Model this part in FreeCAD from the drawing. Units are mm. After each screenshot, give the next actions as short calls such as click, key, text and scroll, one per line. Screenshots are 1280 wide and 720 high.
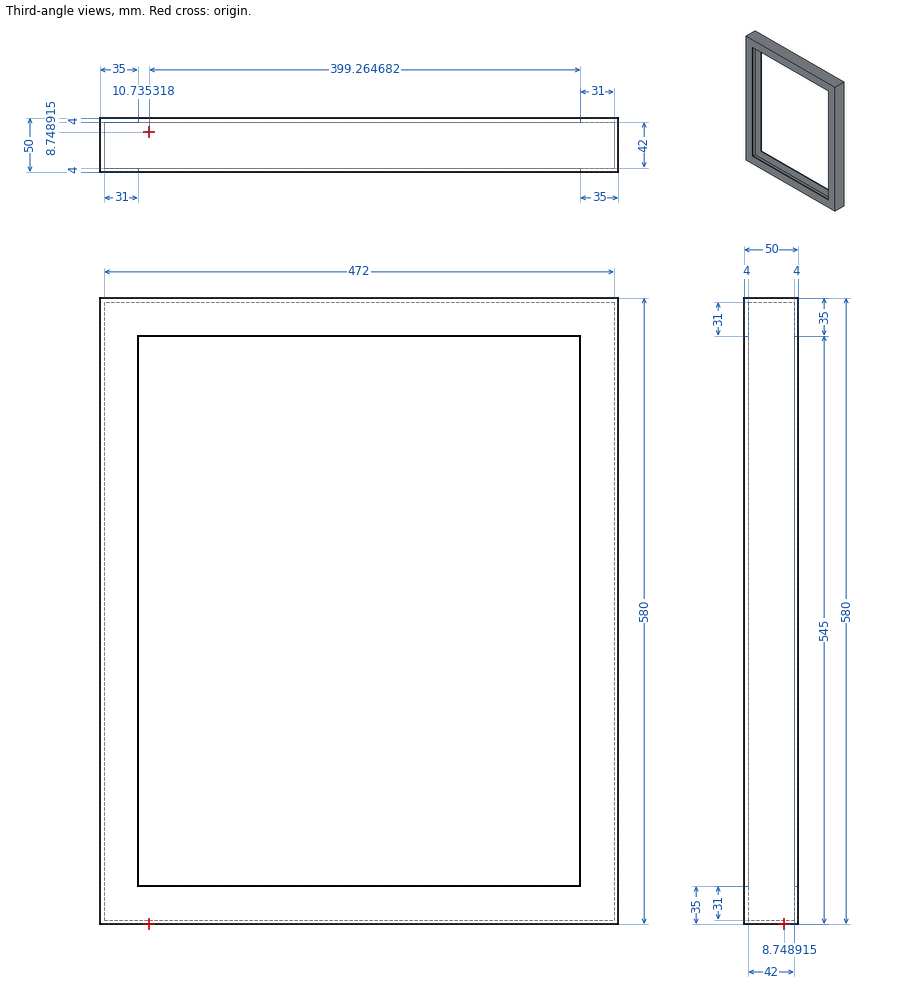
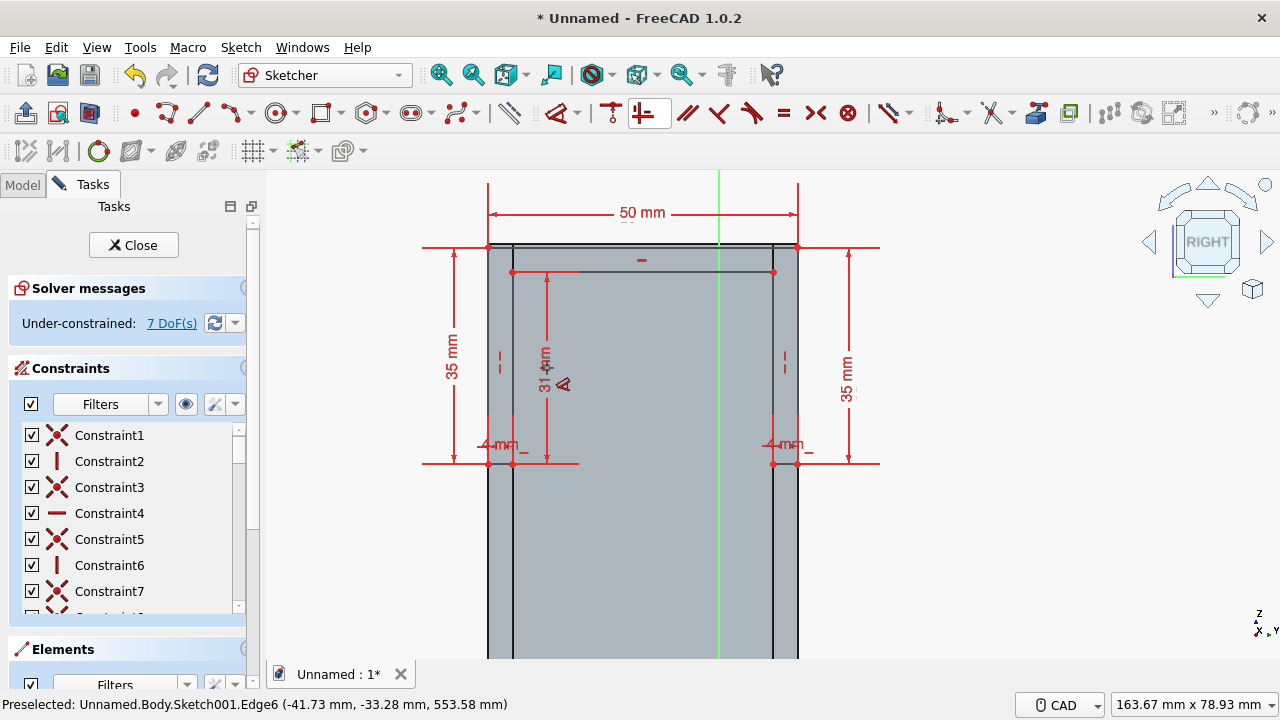
scroll(711, 252, down, 12)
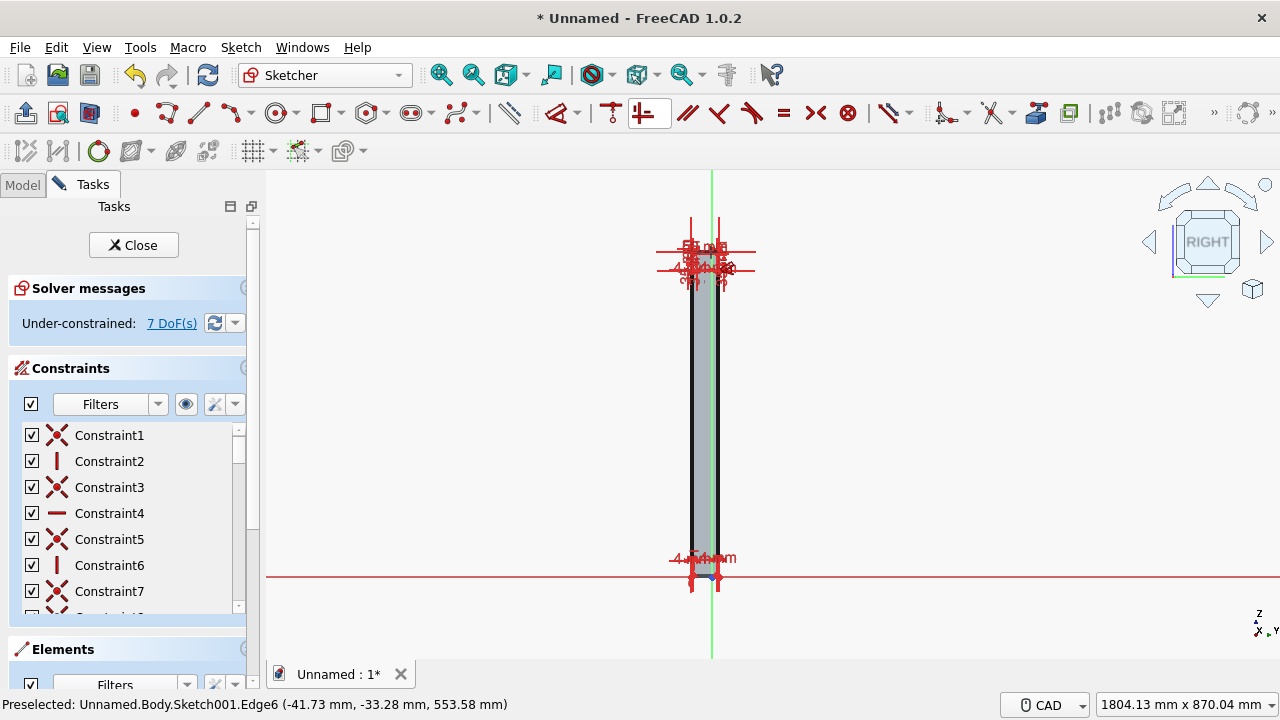
scroll(710, 575, up, 10)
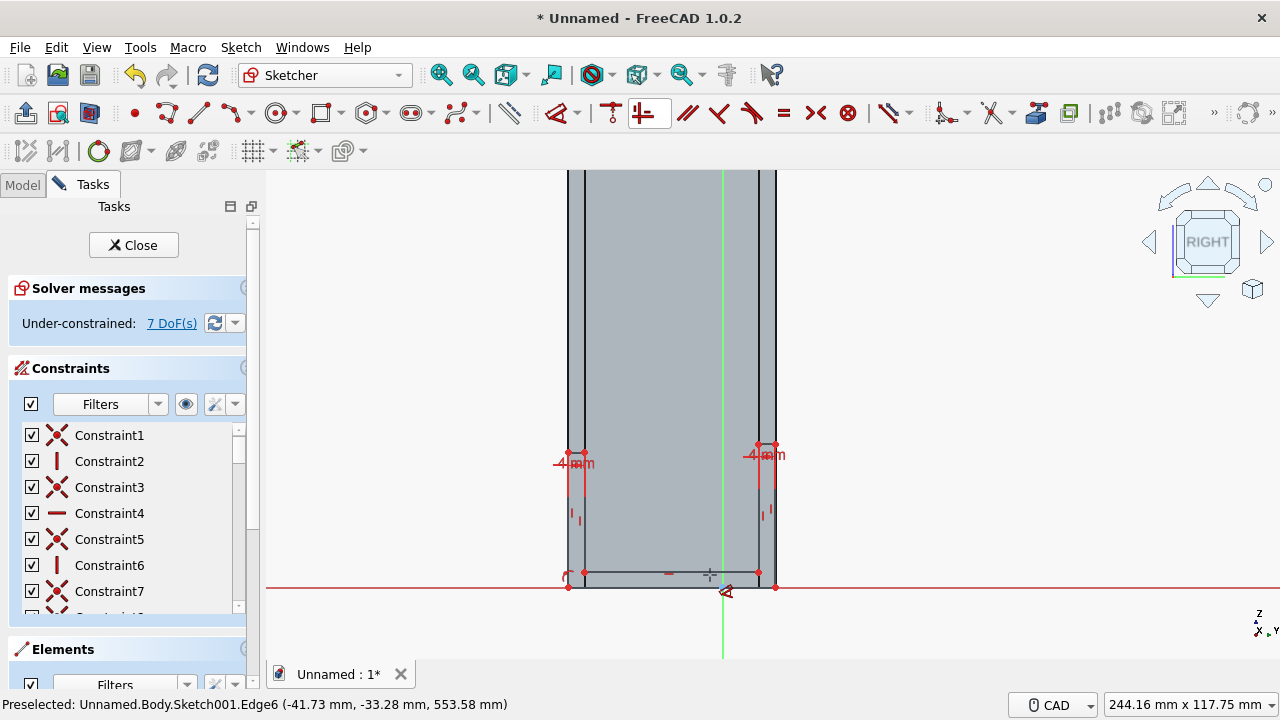
click(707, 572)
click(672, 606)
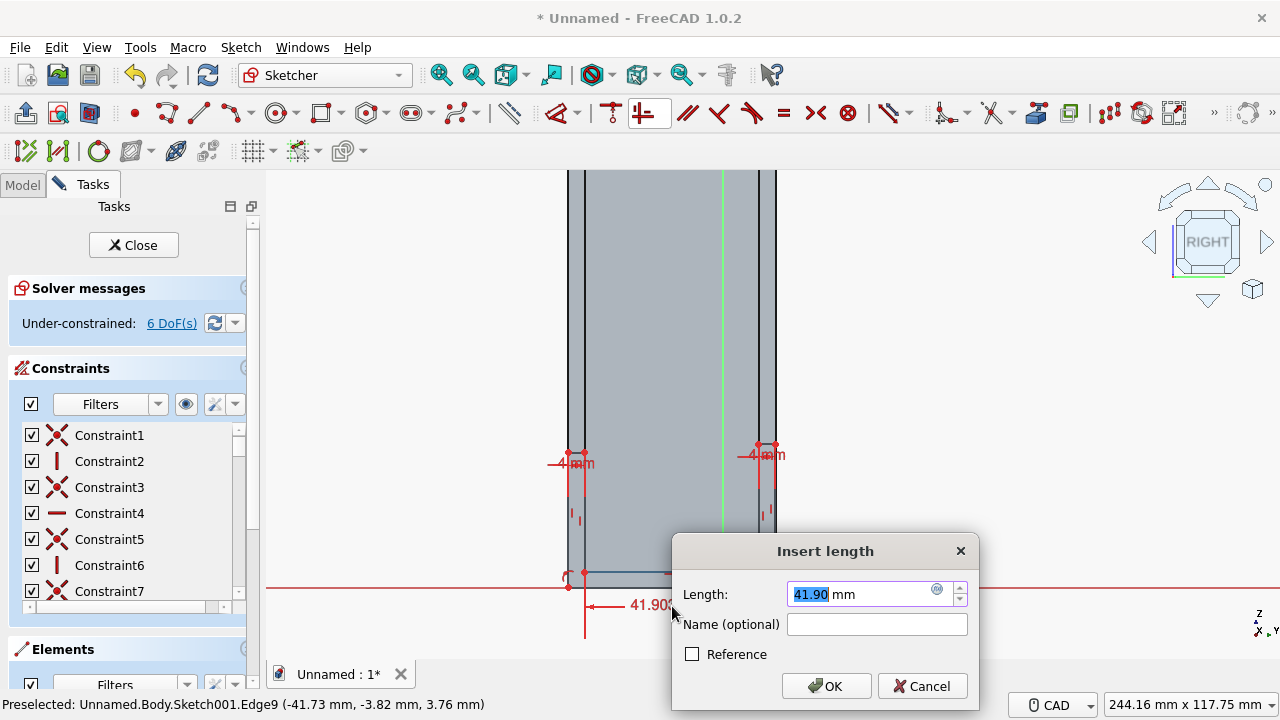
text(42)
key(Return)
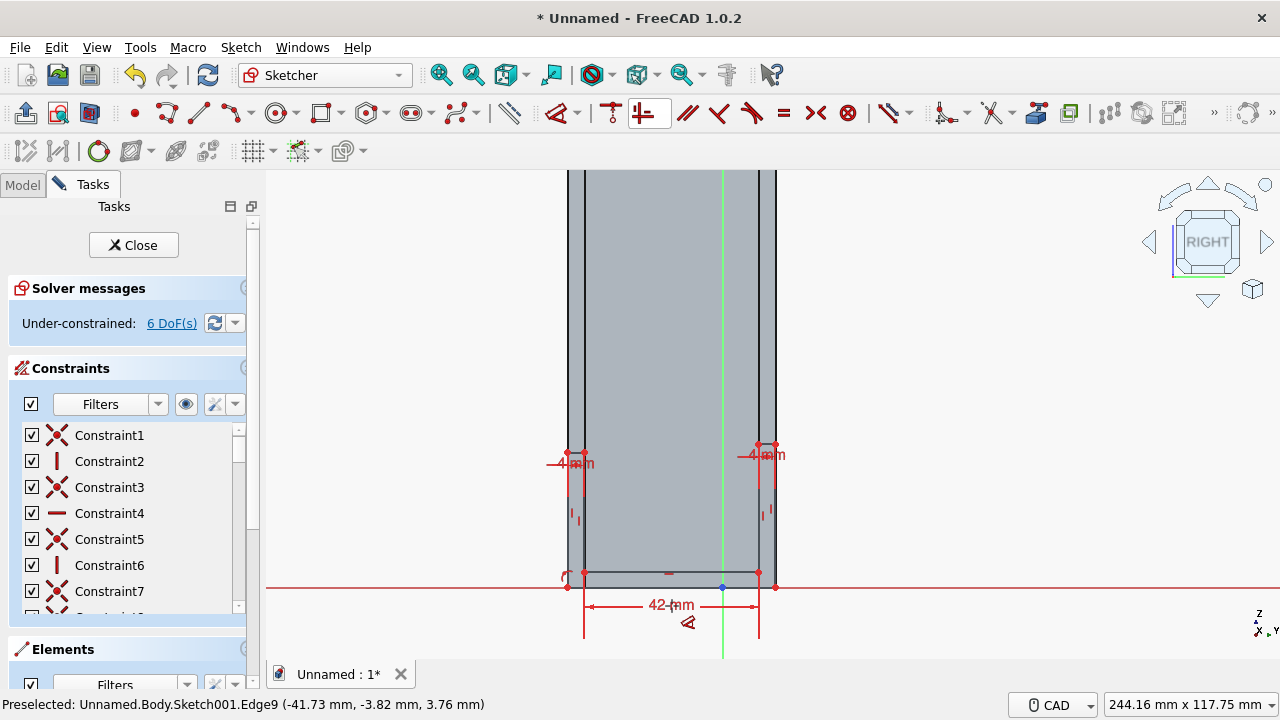
click(584, 536)
click(550, 512)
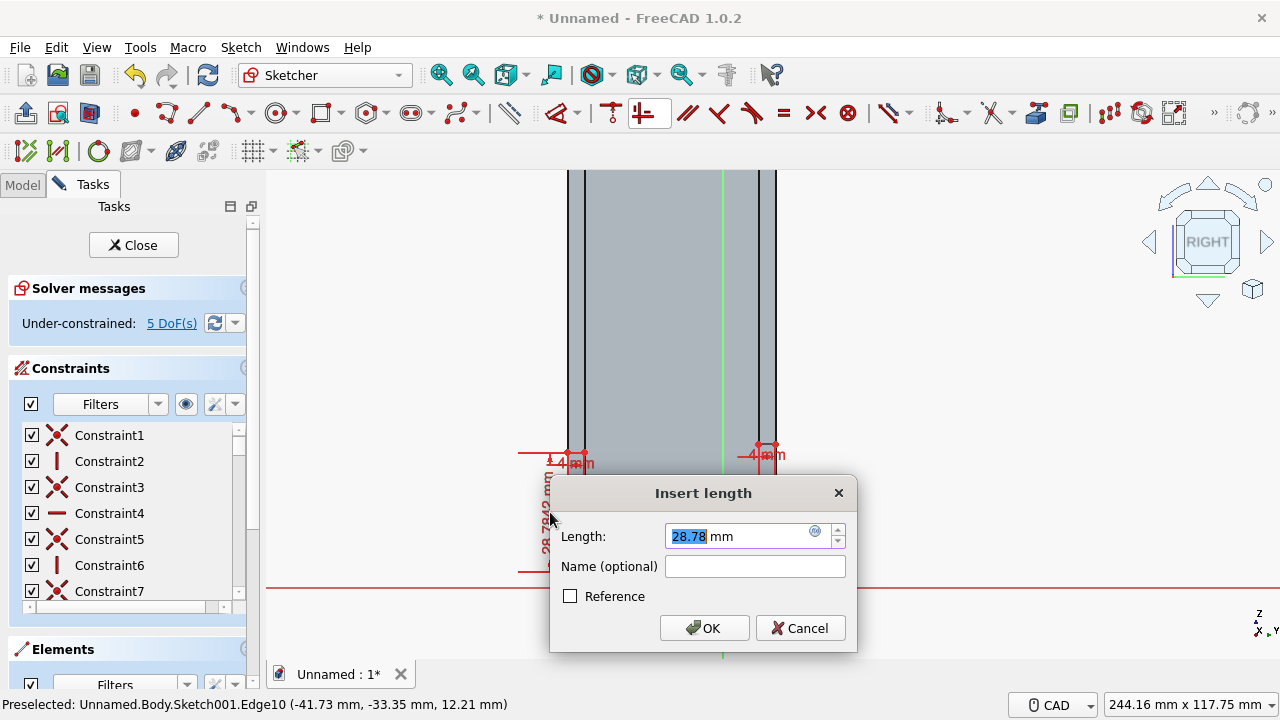
text(31)
key(Return)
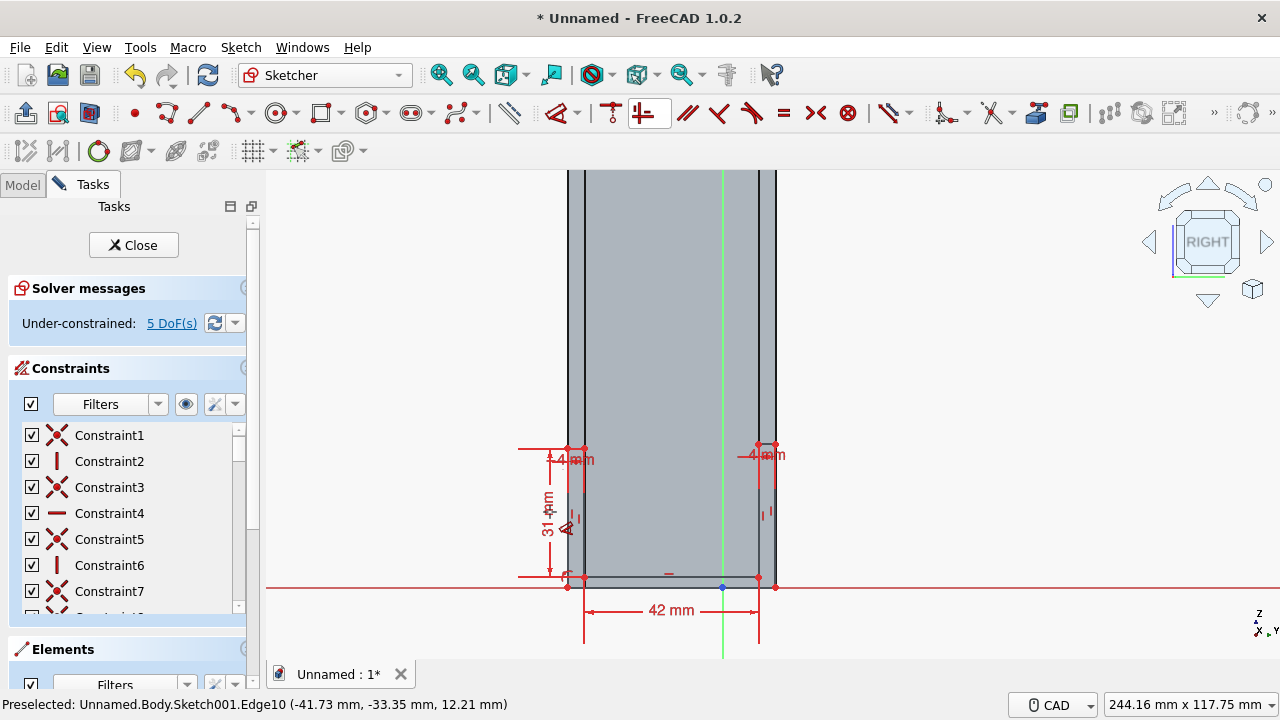
click(568, 490)
click(534, 486)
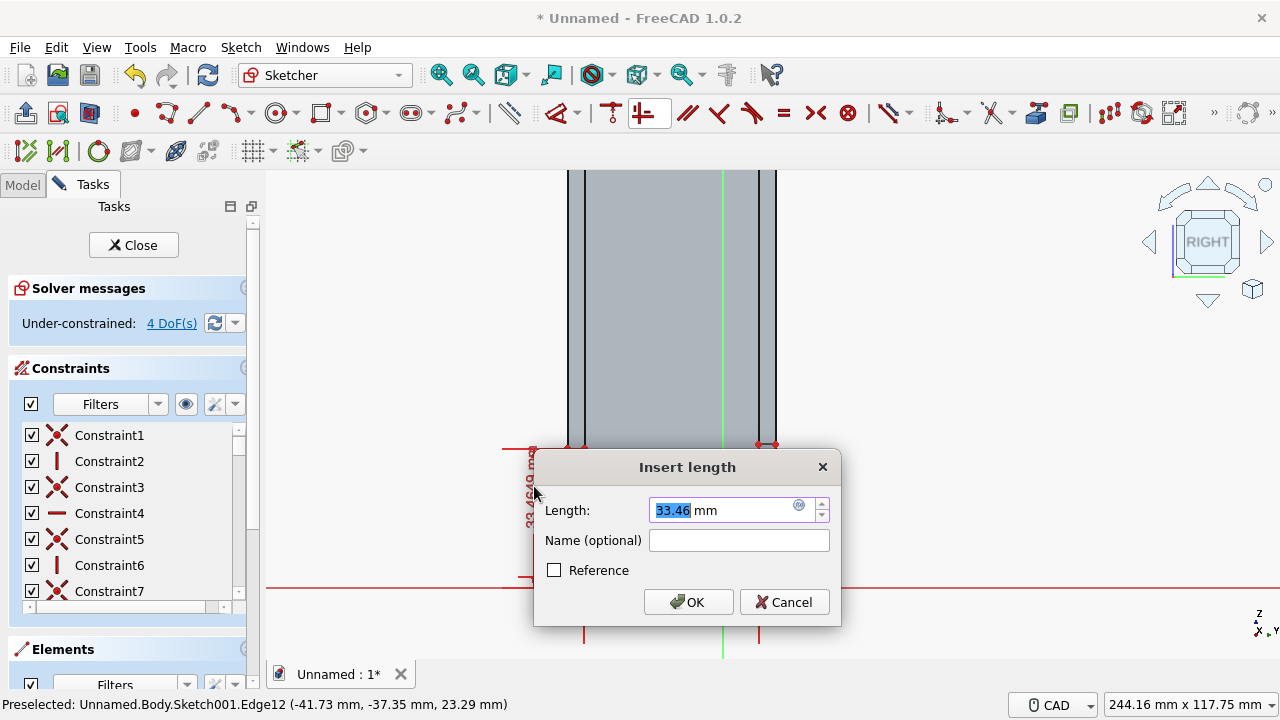
text(35)
key(Return)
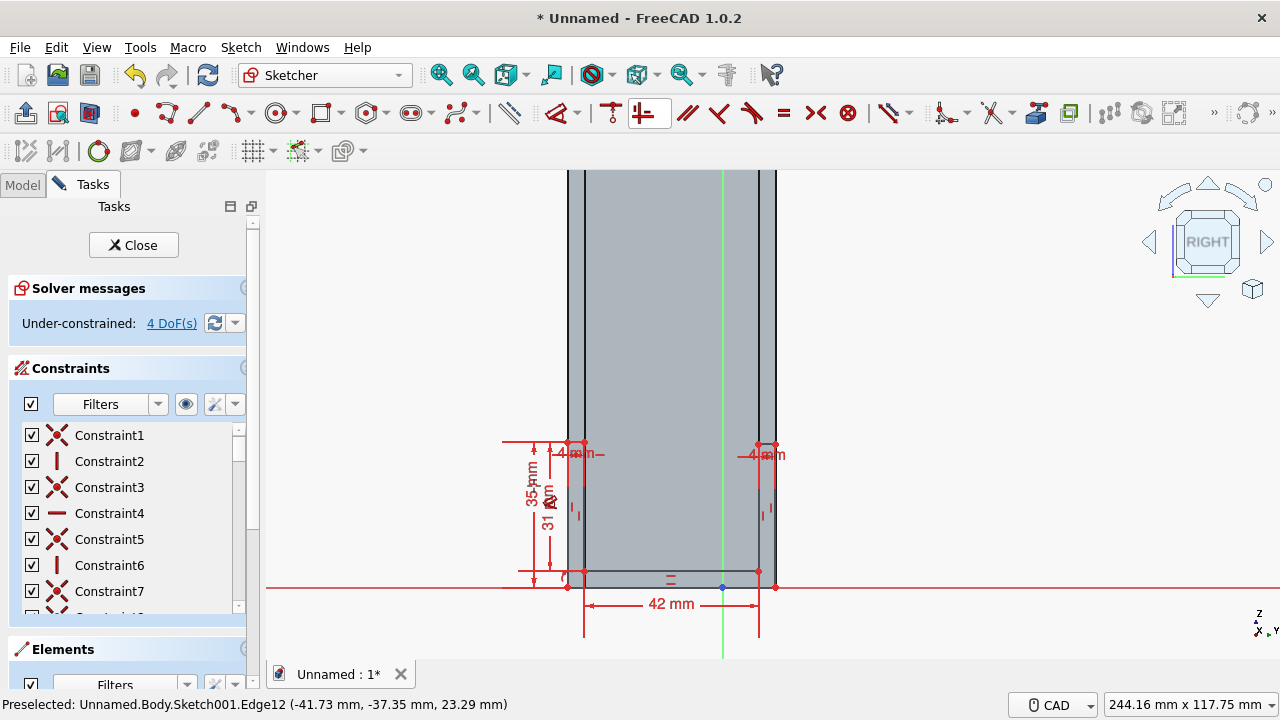
click(775, 545)
click(809, 516)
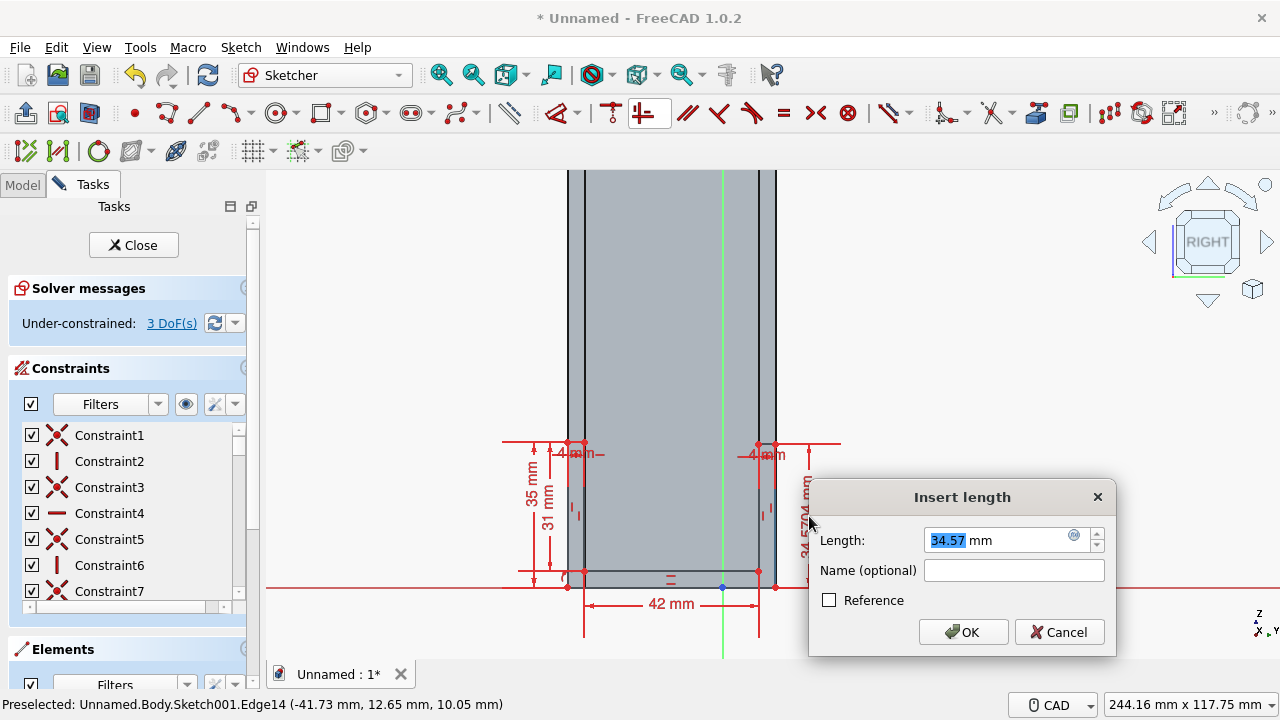
text(35)
key(Return)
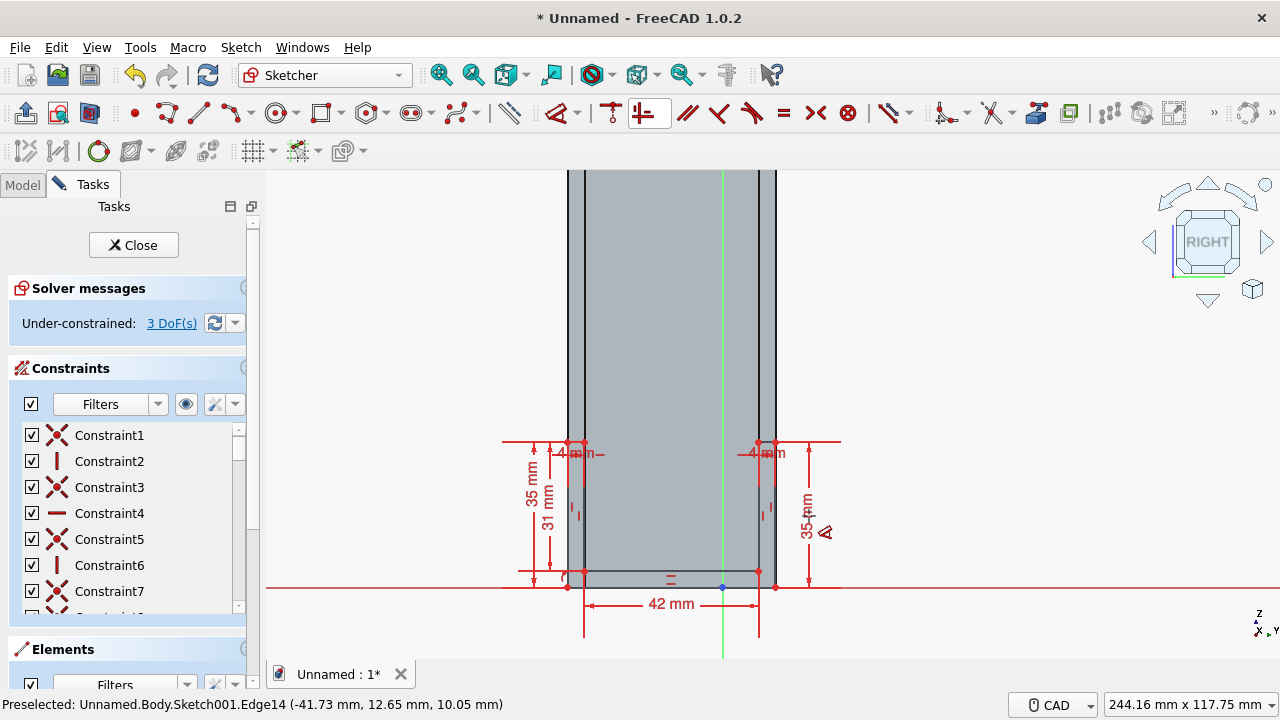
scroll(710, 576, down, 10)